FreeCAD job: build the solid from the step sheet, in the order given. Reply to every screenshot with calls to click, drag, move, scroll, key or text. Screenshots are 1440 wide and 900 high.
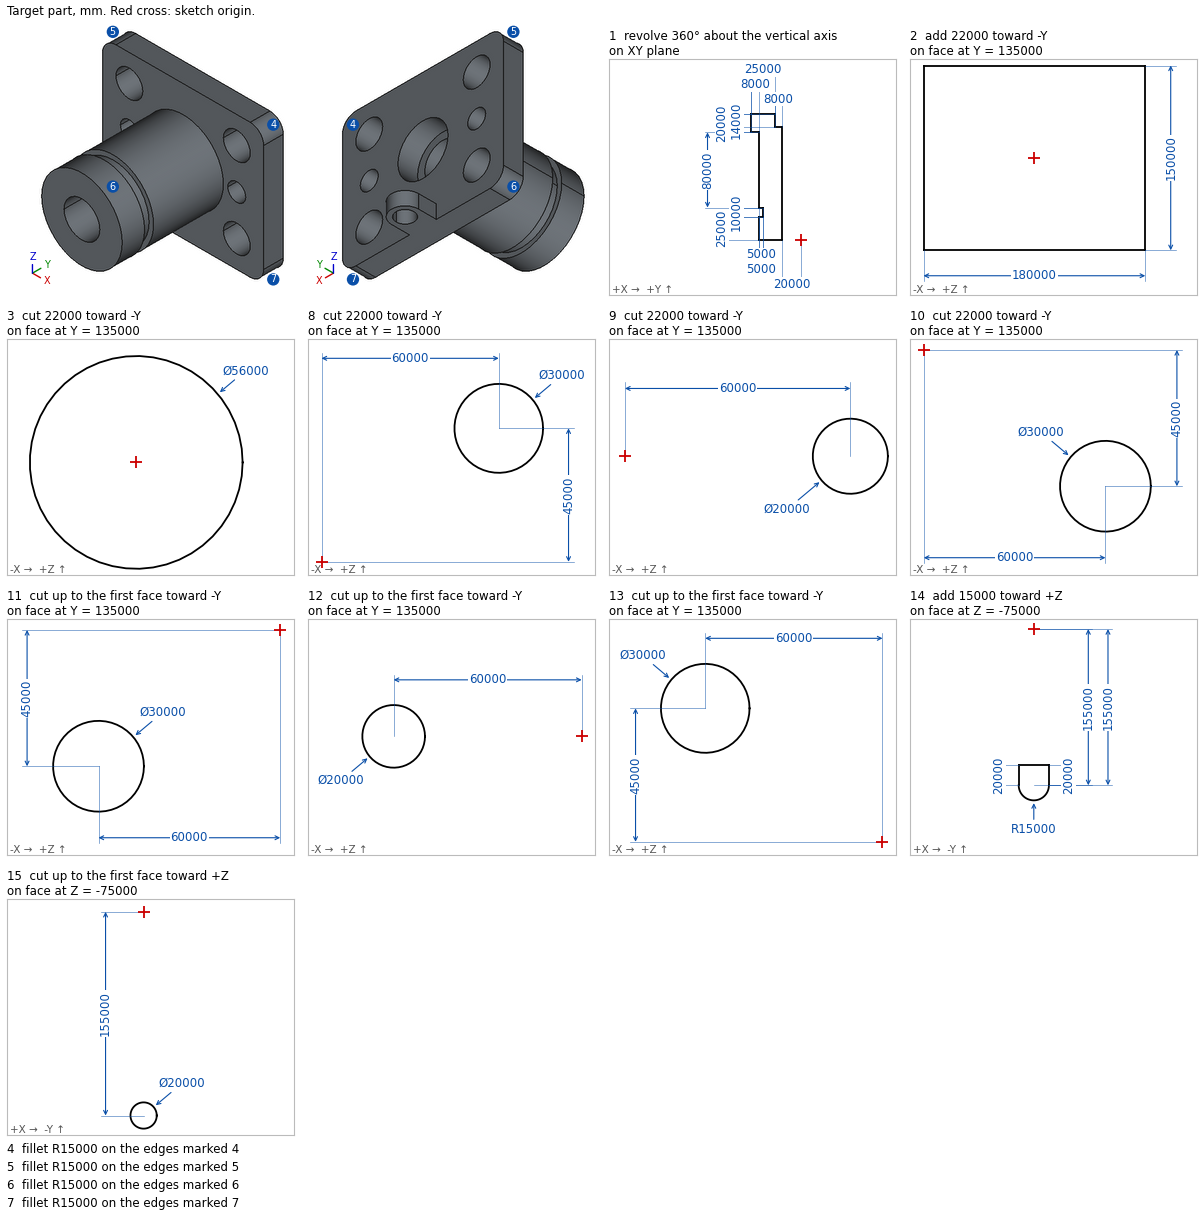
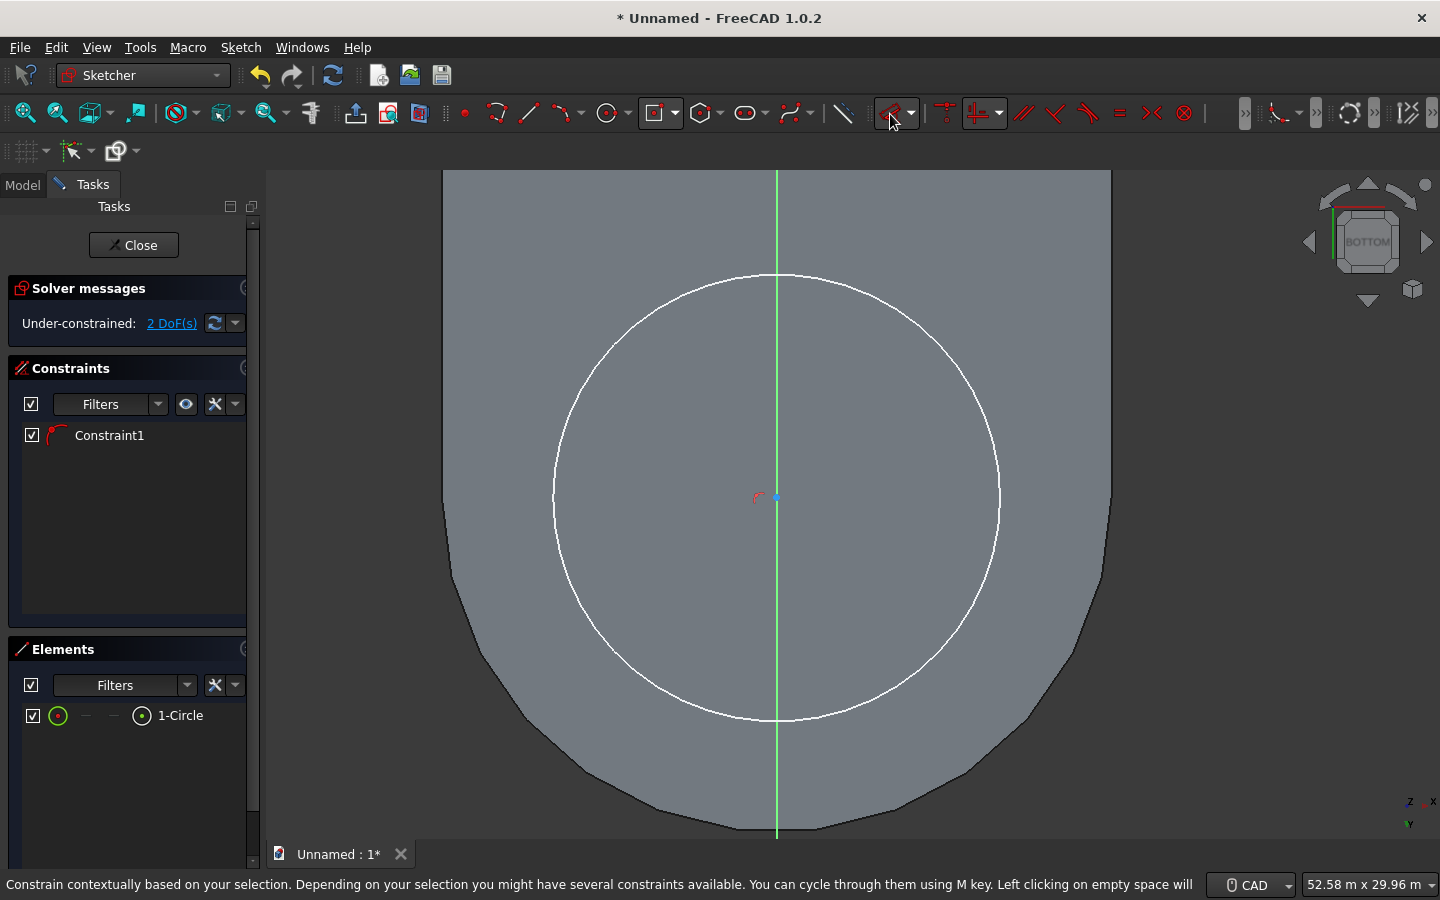
click(934, 340)
click(957, 317)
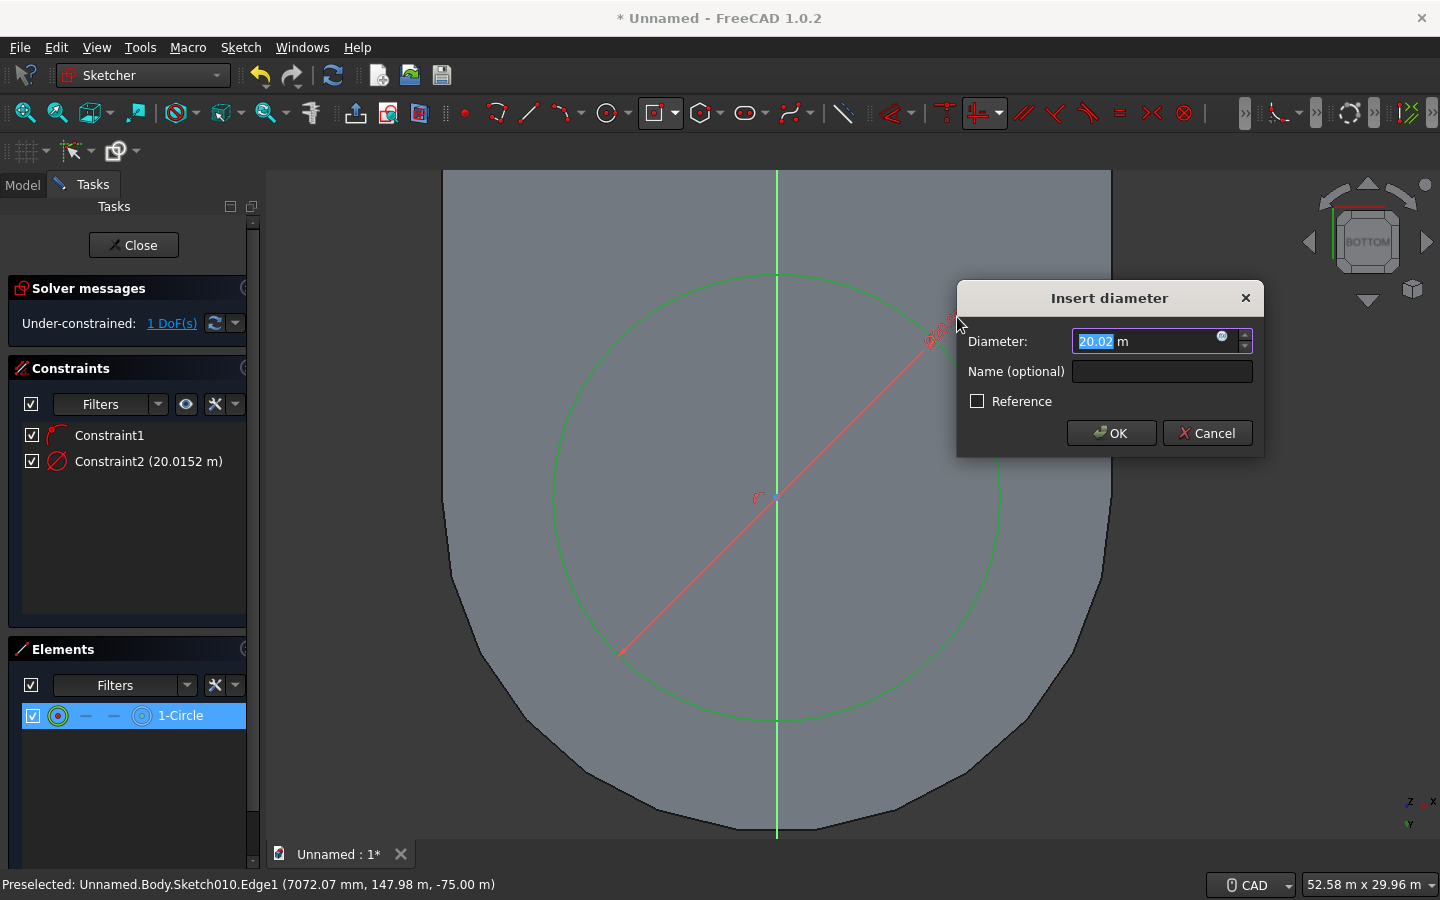
key(ctrl+a)
text(20000 mm)
key(Return)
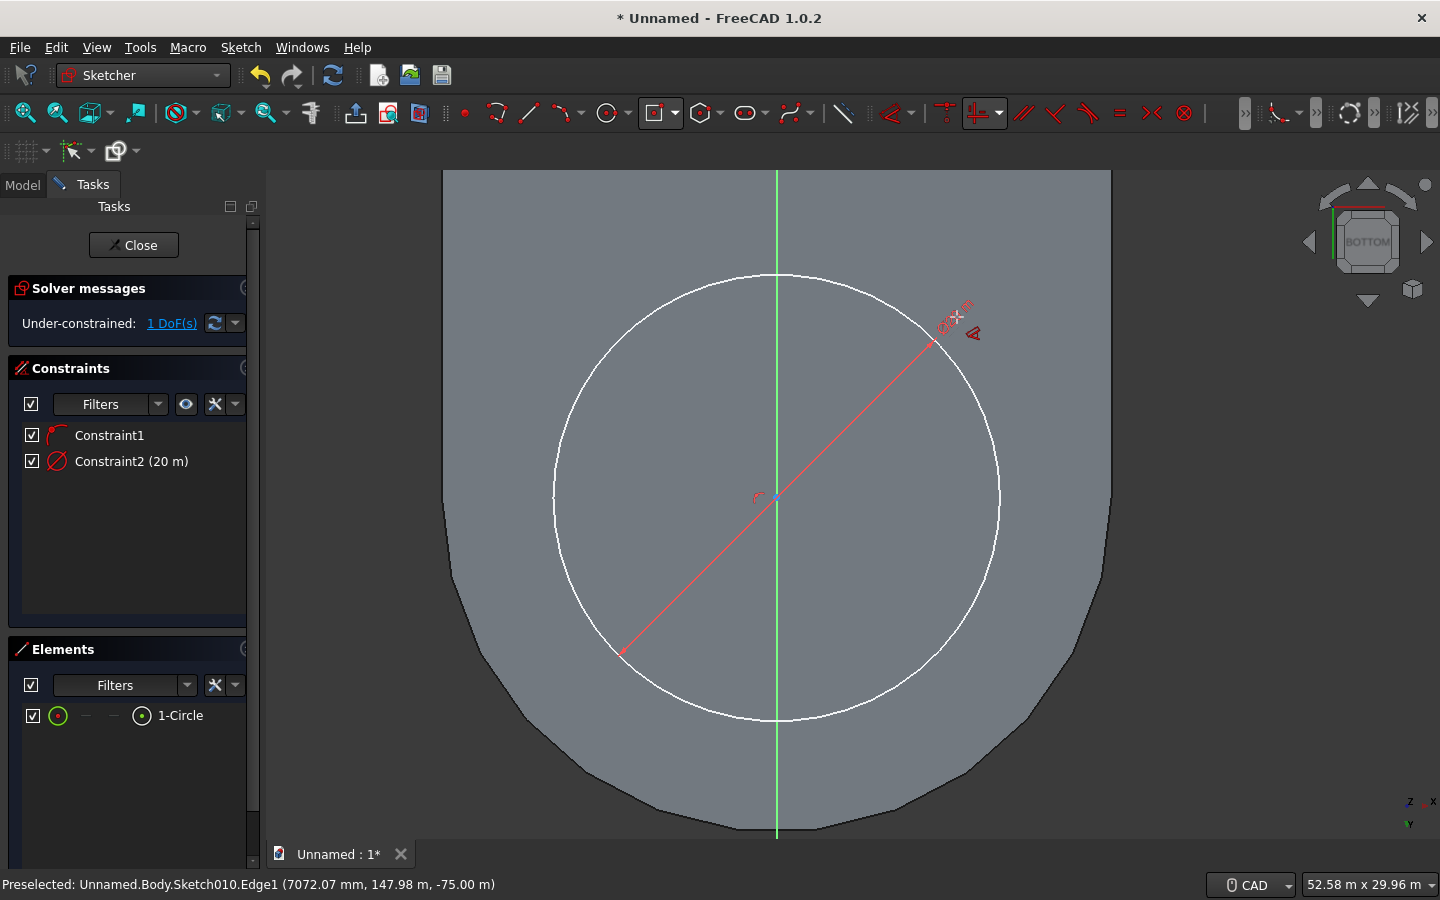
click(777, 498)
click(811, 348)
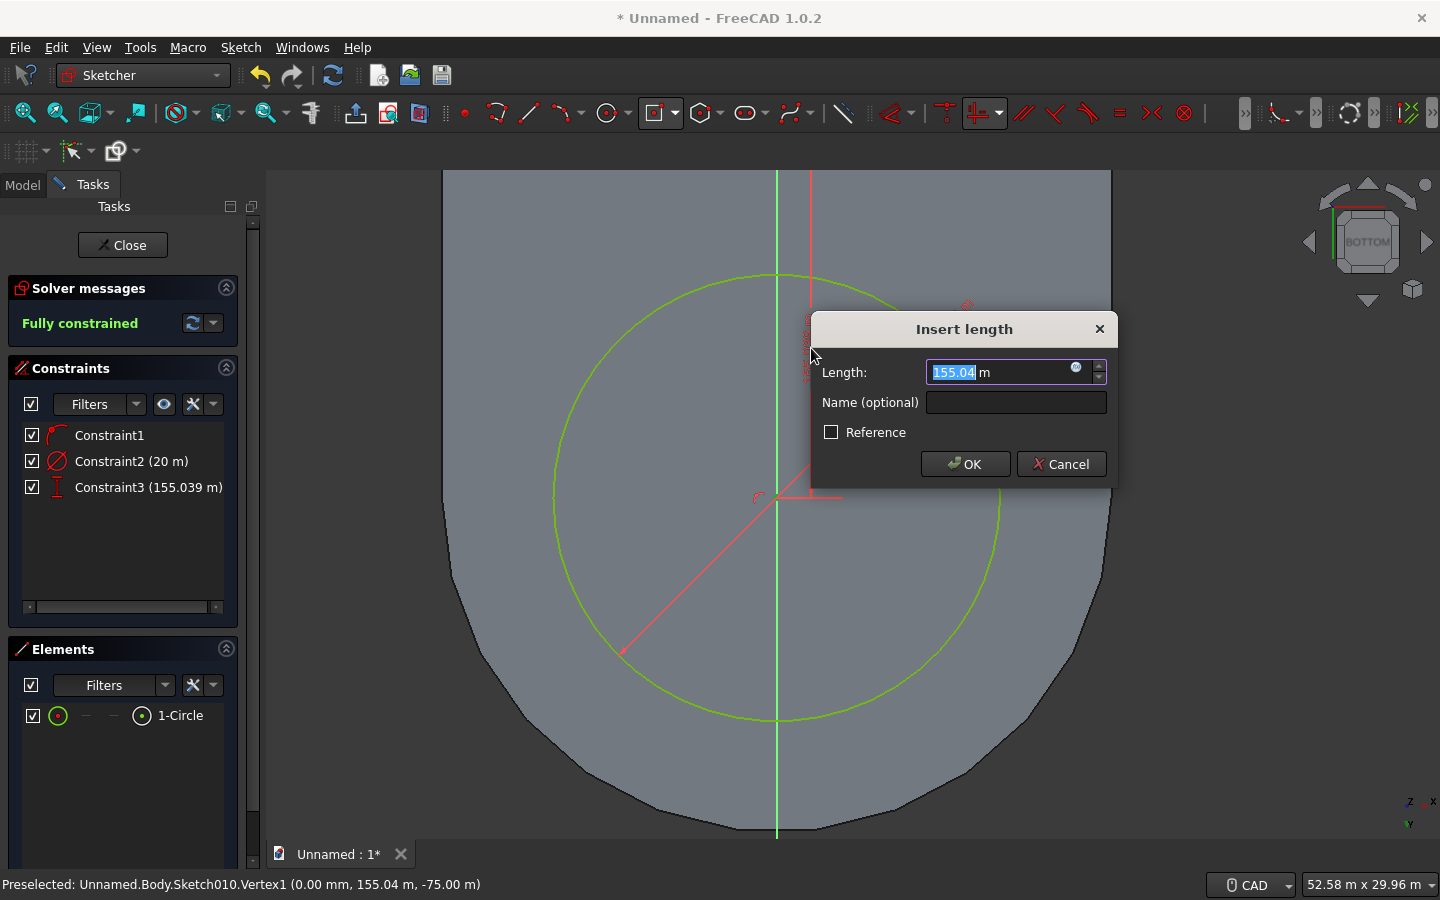
key(ctrl+a)
text(155000 mm)
key(Return)
key(Escape)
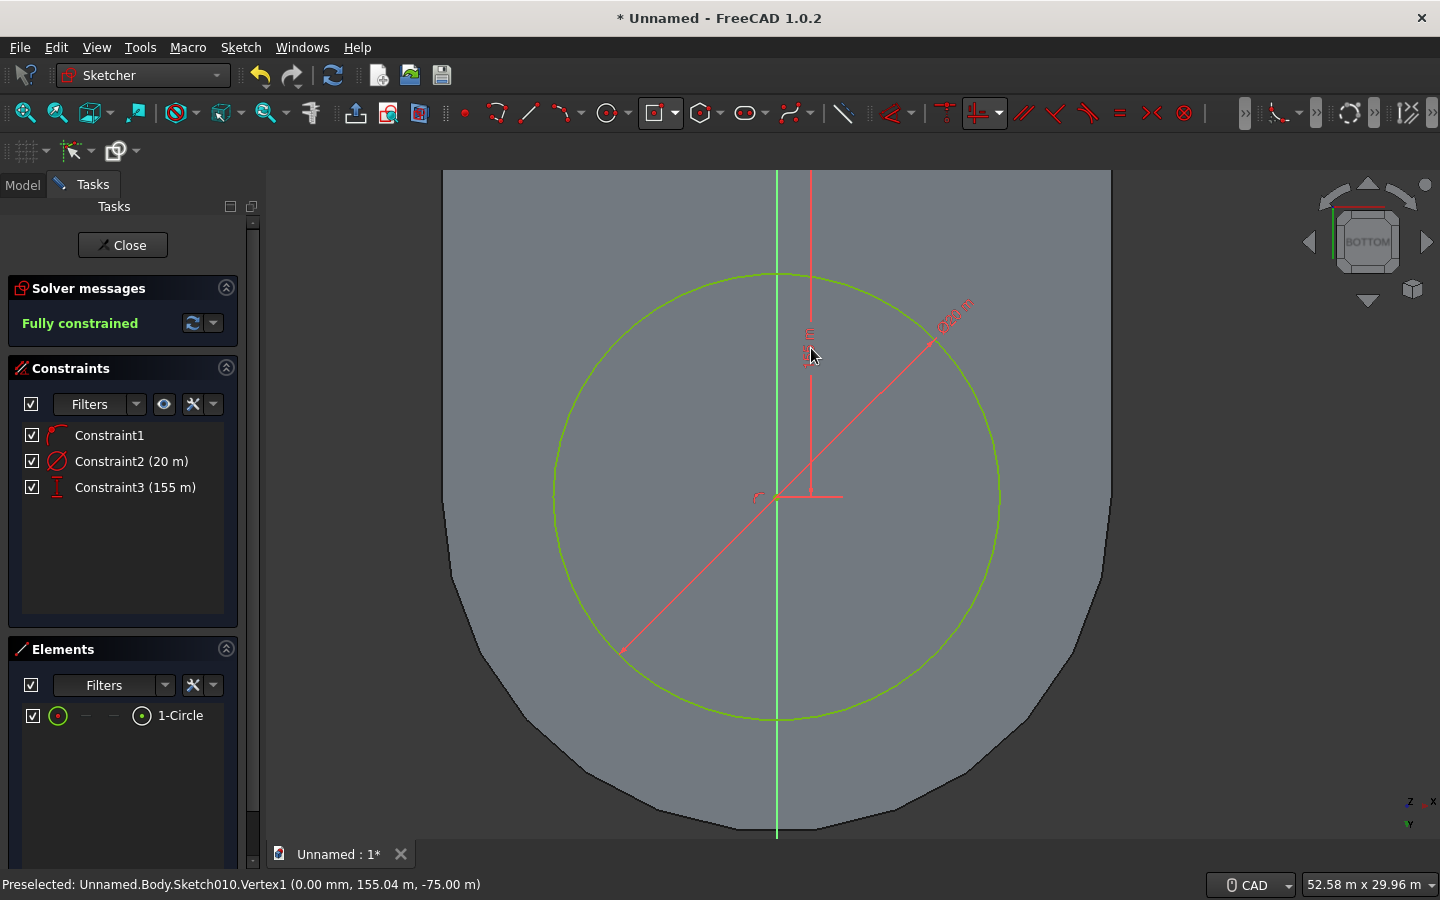
click(123, 245)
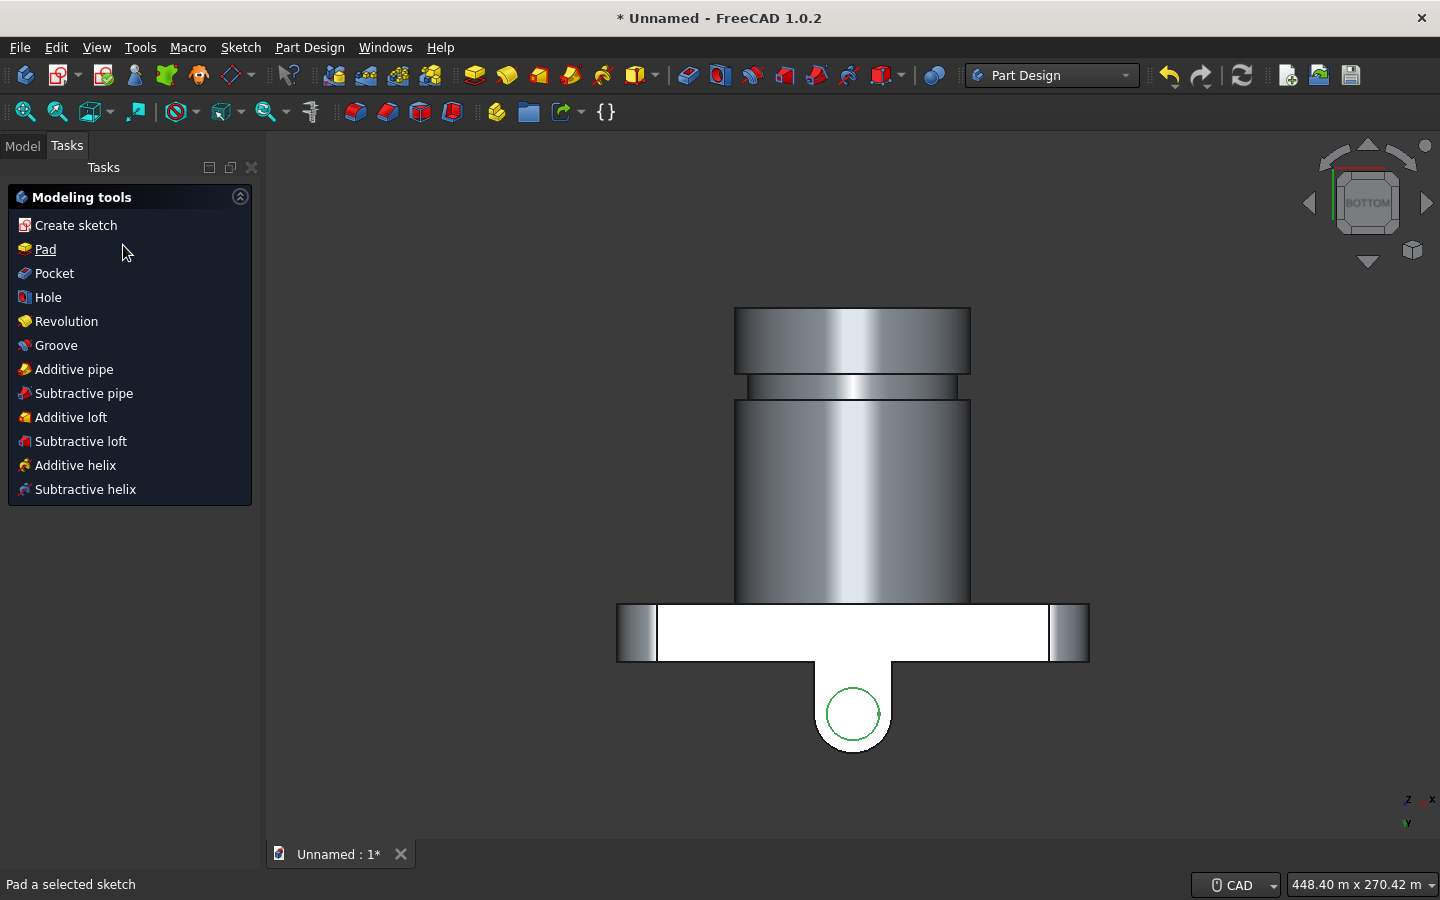
click(690, 76)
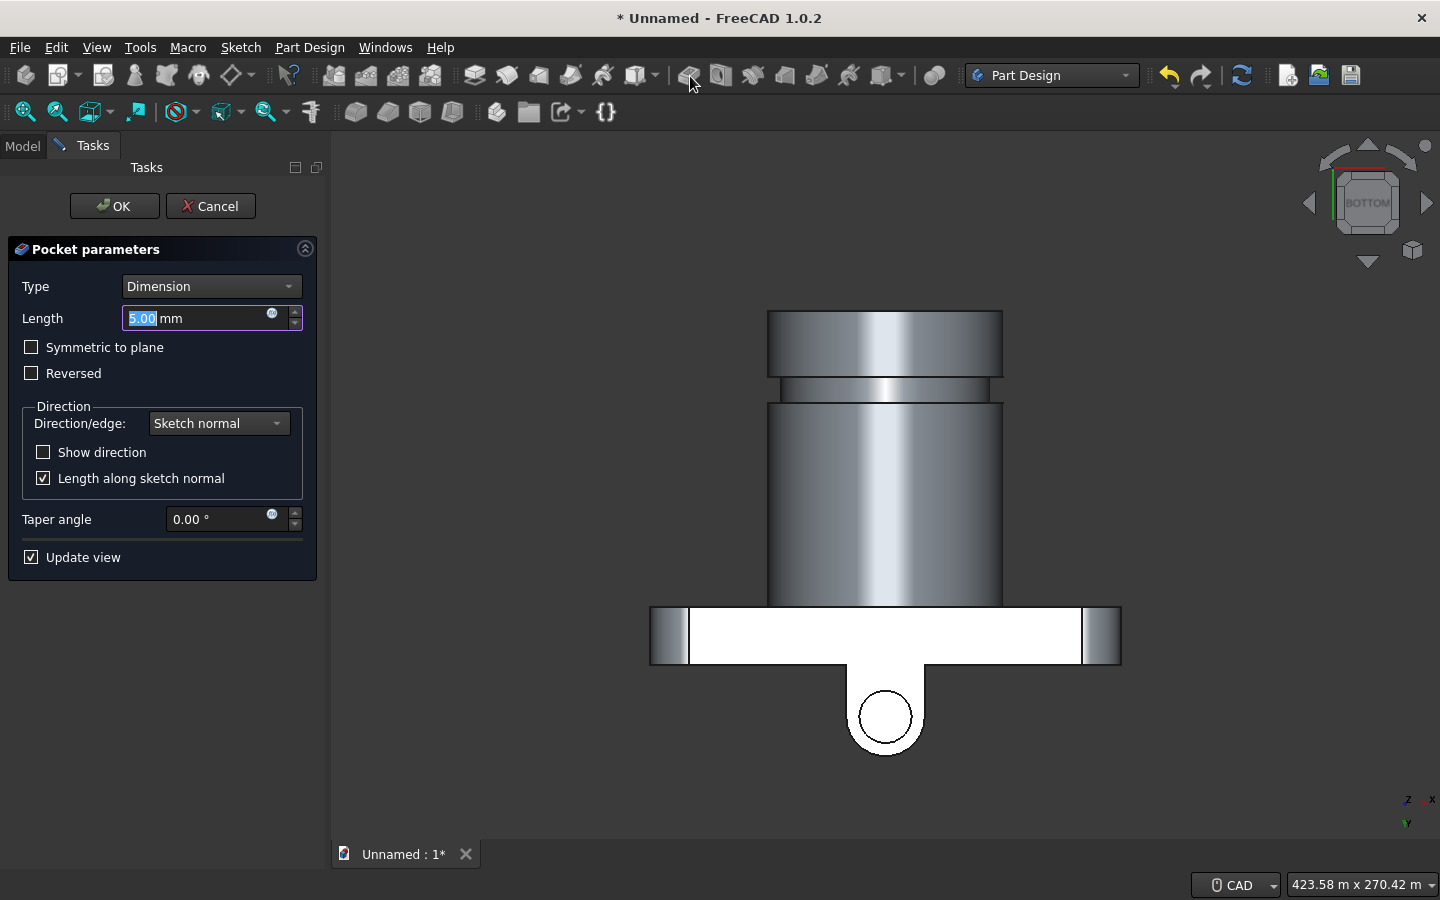
click(212, 286)